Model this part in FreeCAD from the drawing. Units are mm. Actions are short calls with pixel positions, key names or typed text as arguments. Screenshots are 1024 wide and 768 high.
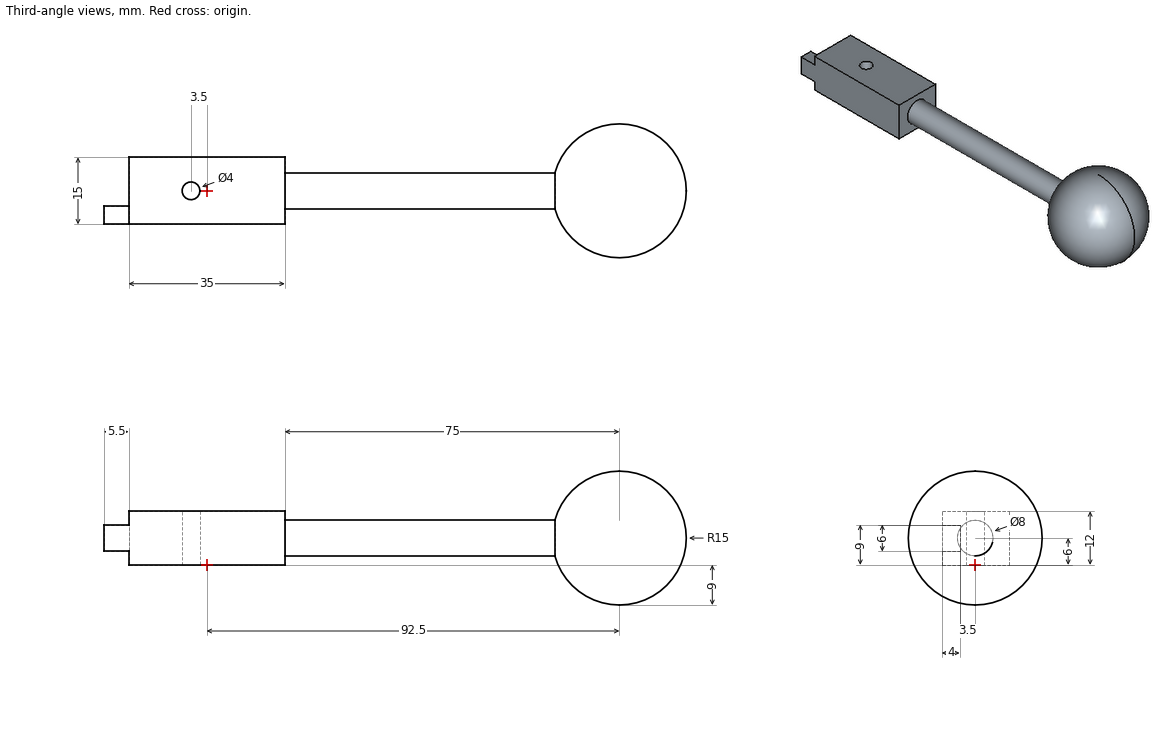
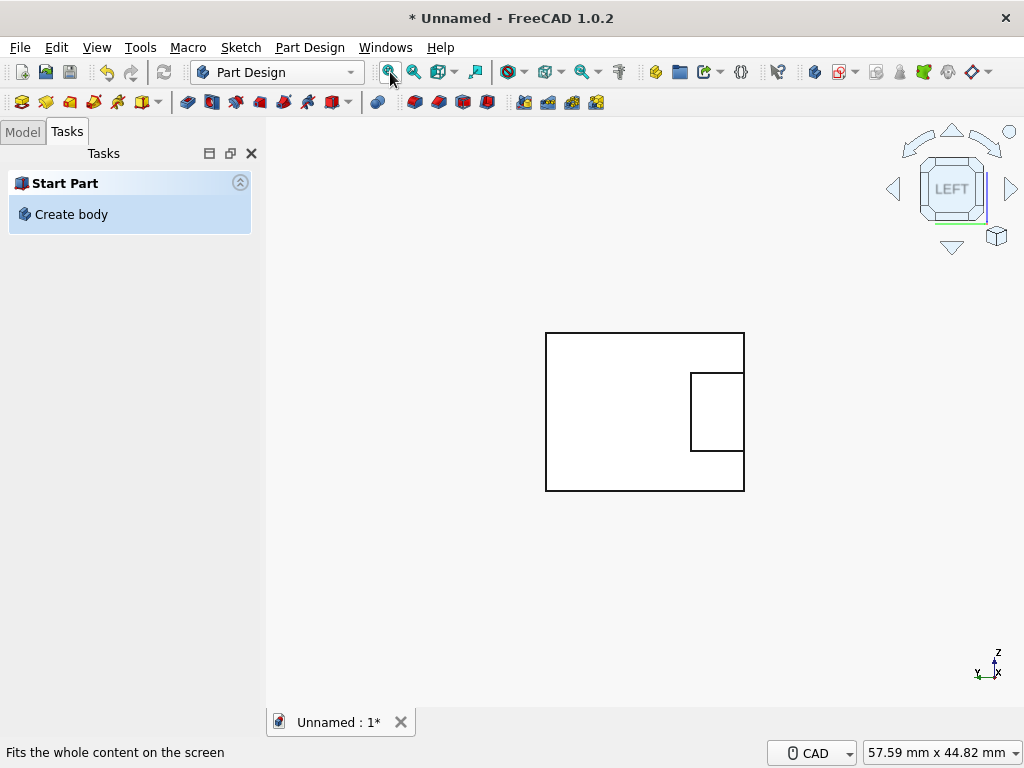
key(0)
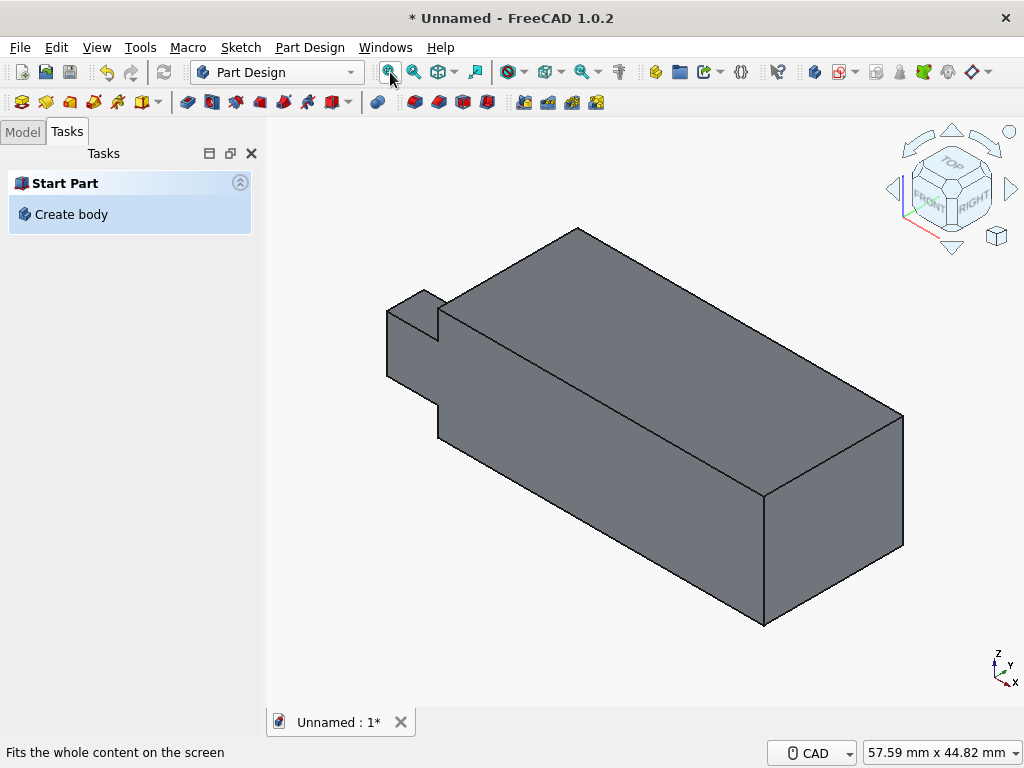
click(833, 520)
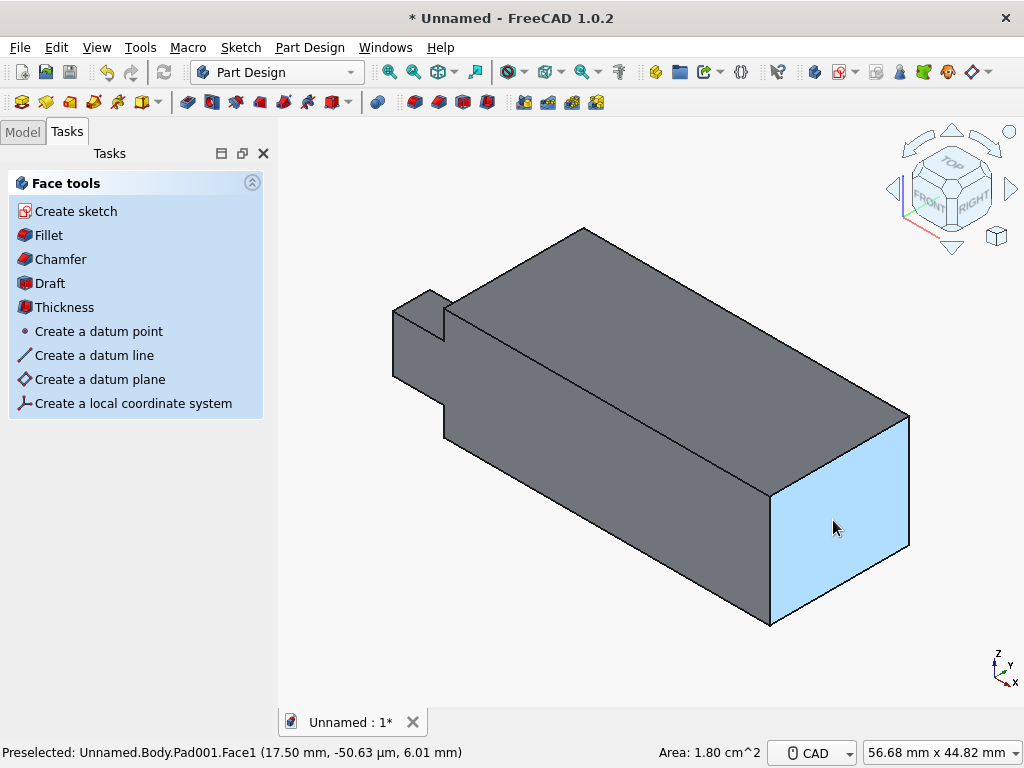
click(840, 72)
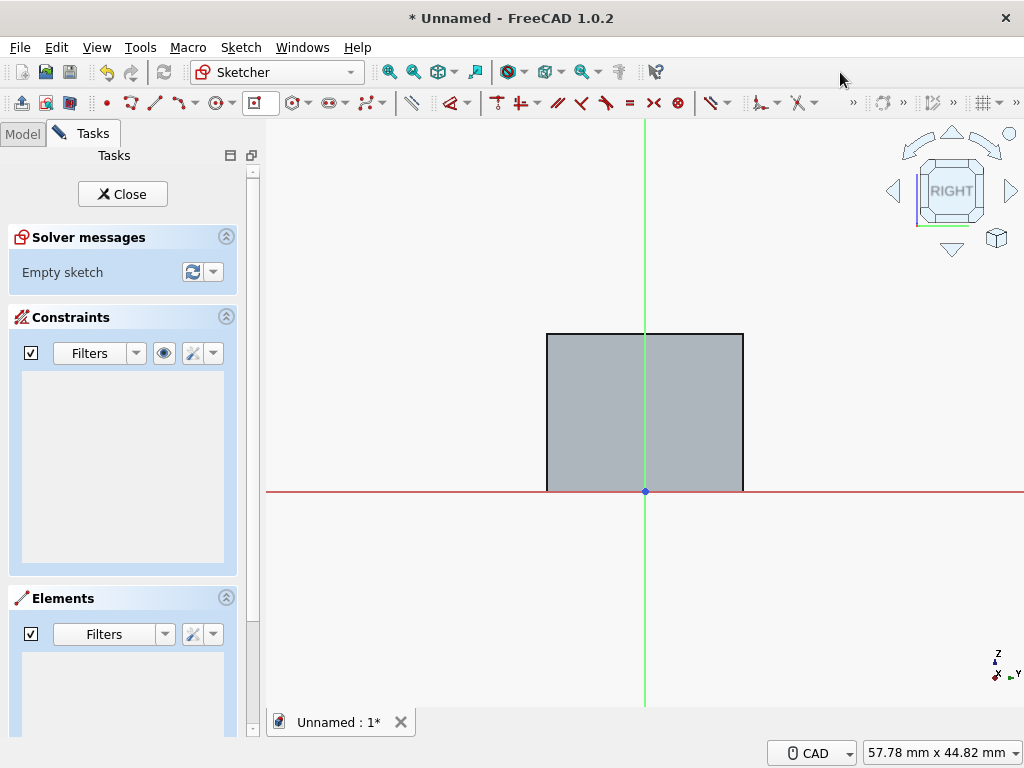
scroll(685, 434, up, 5)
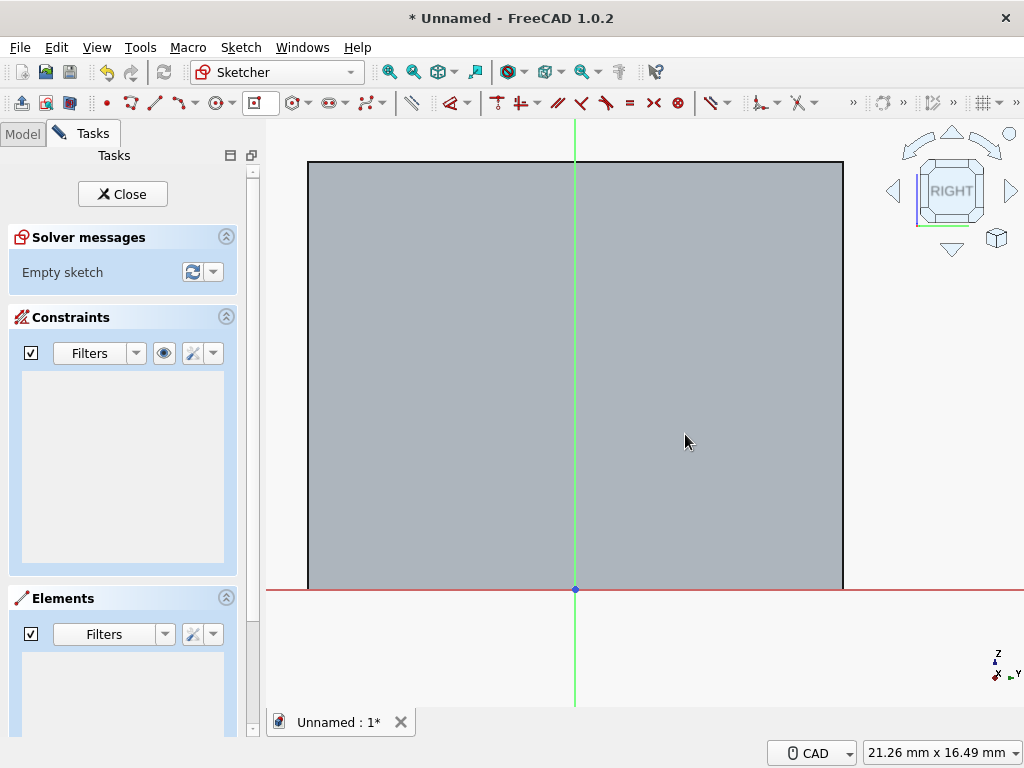
click(216, 104)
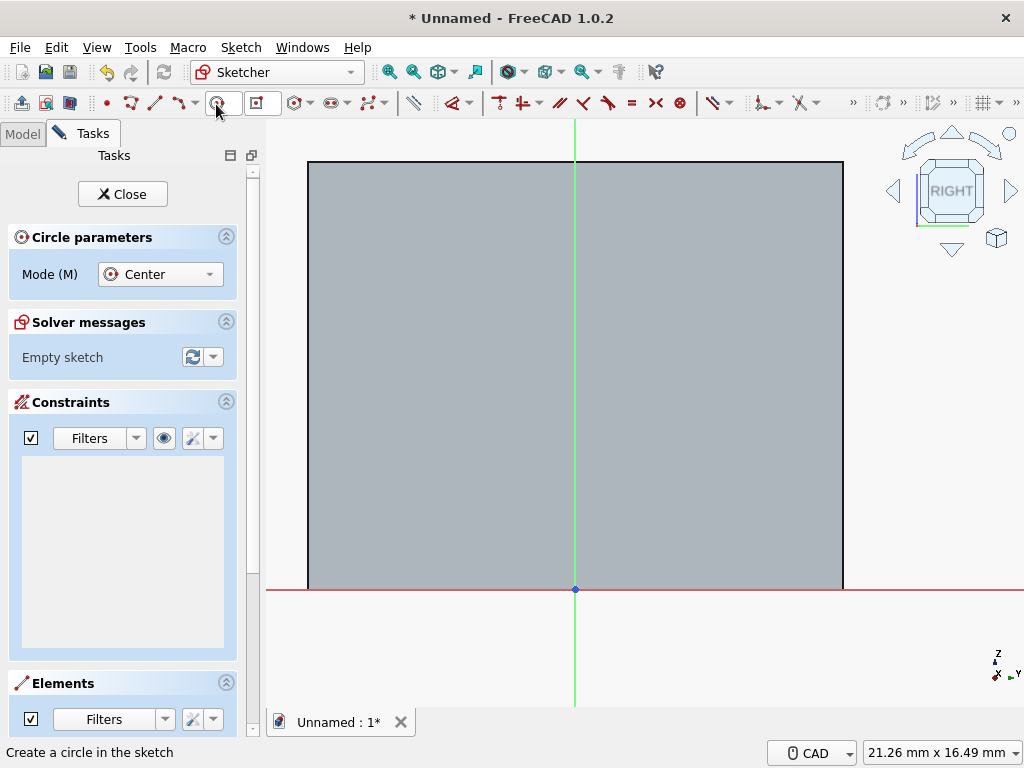
click(575, 376)
click(676, 275)
key(Escape)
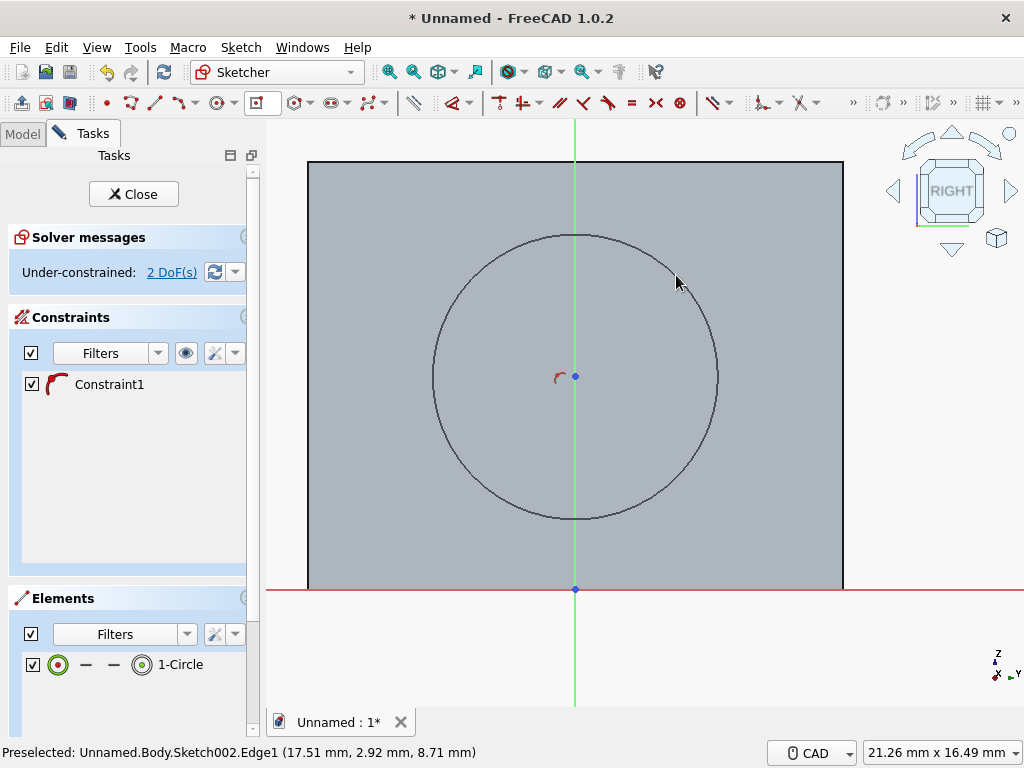
click(452, 104)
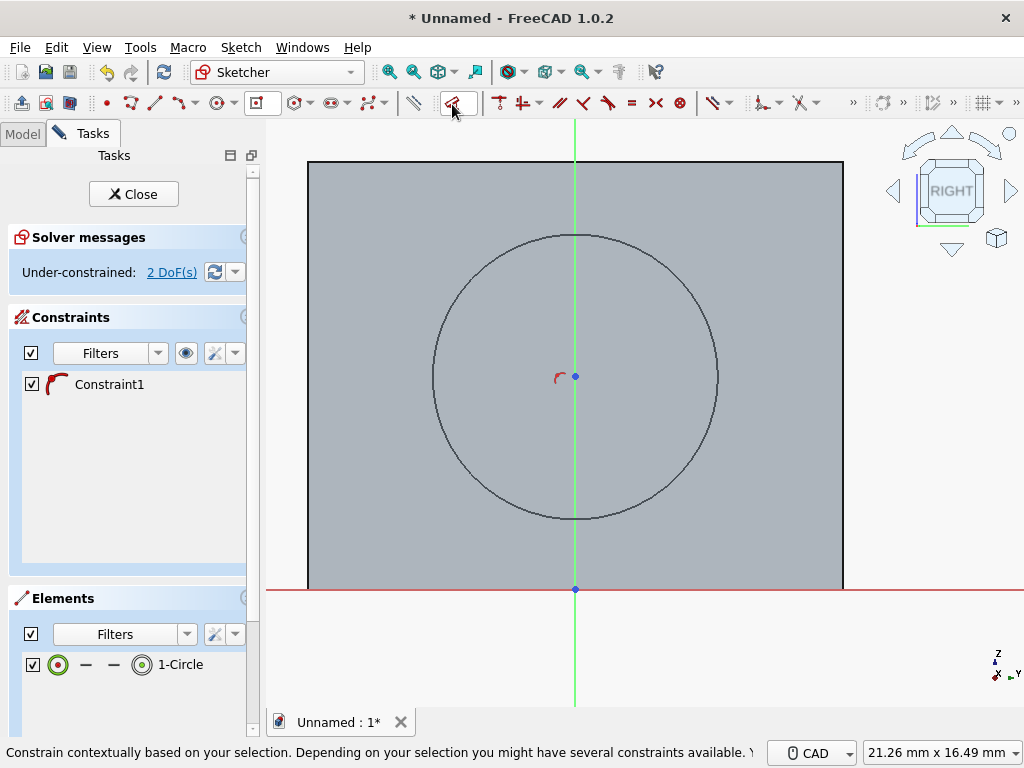
click(676, 276)
click(699, 253)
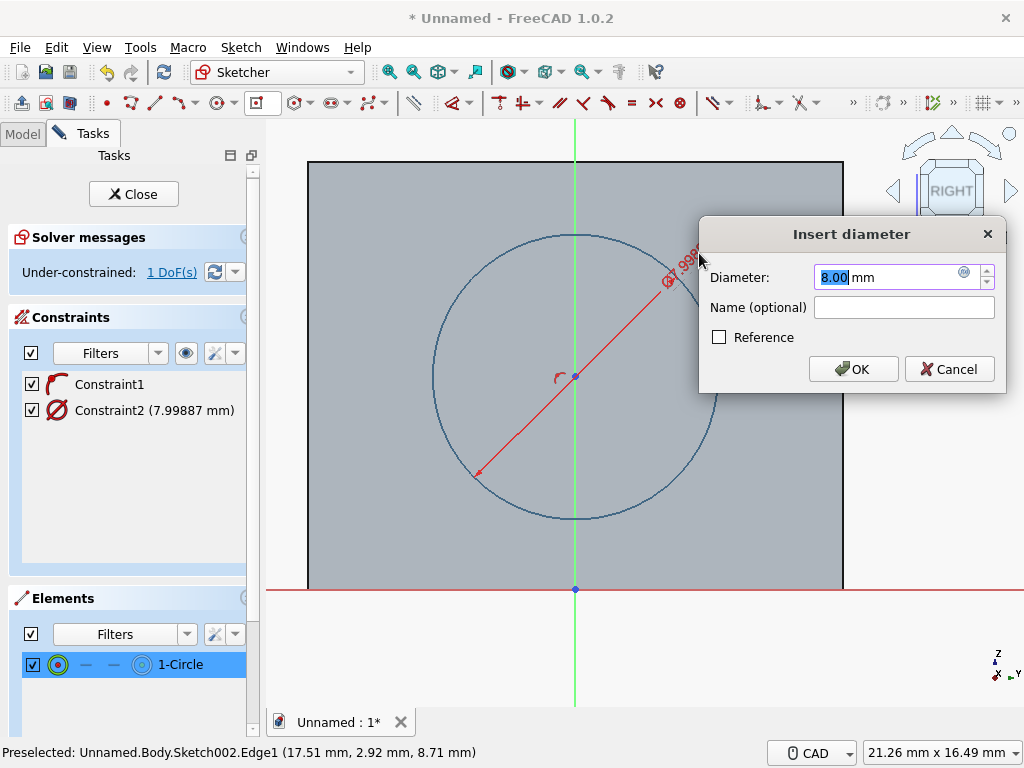
text(8)
key(Return)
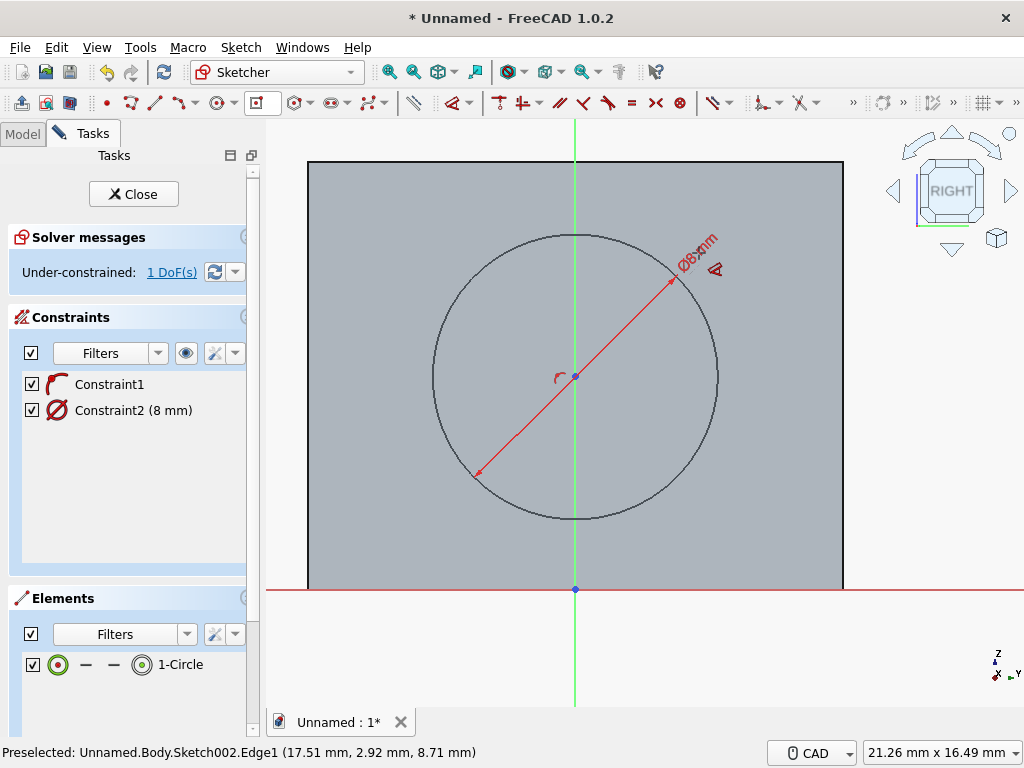
click(575, 377)
click(609, 483)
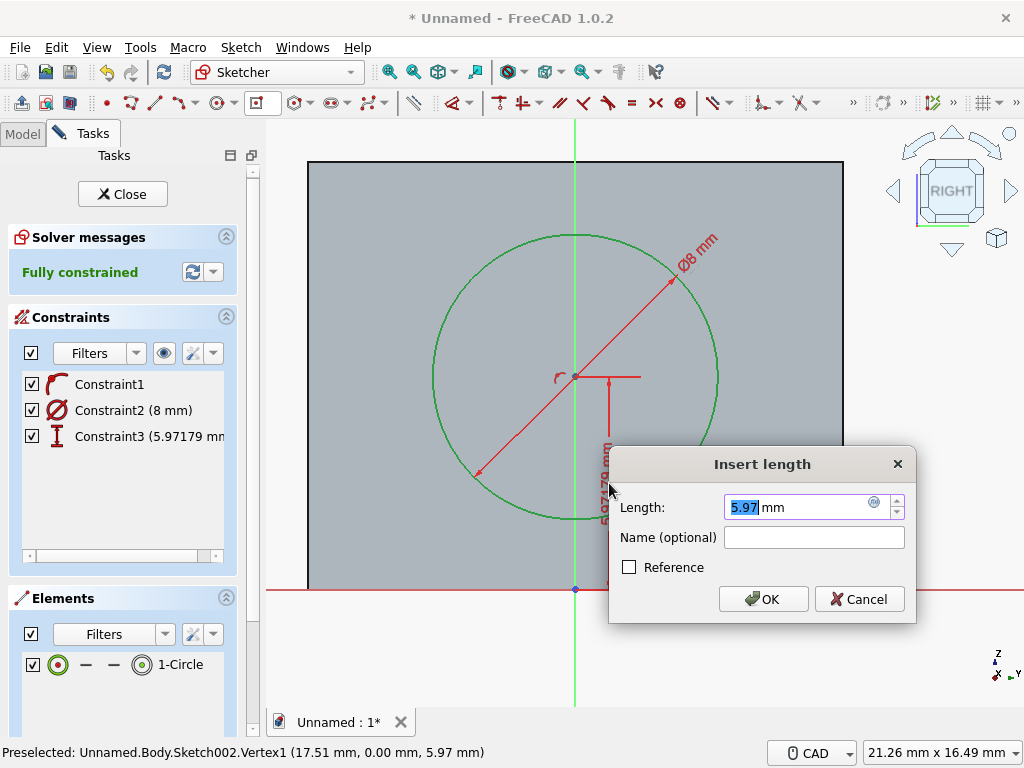
text(6)
key(Return)
key(Escape)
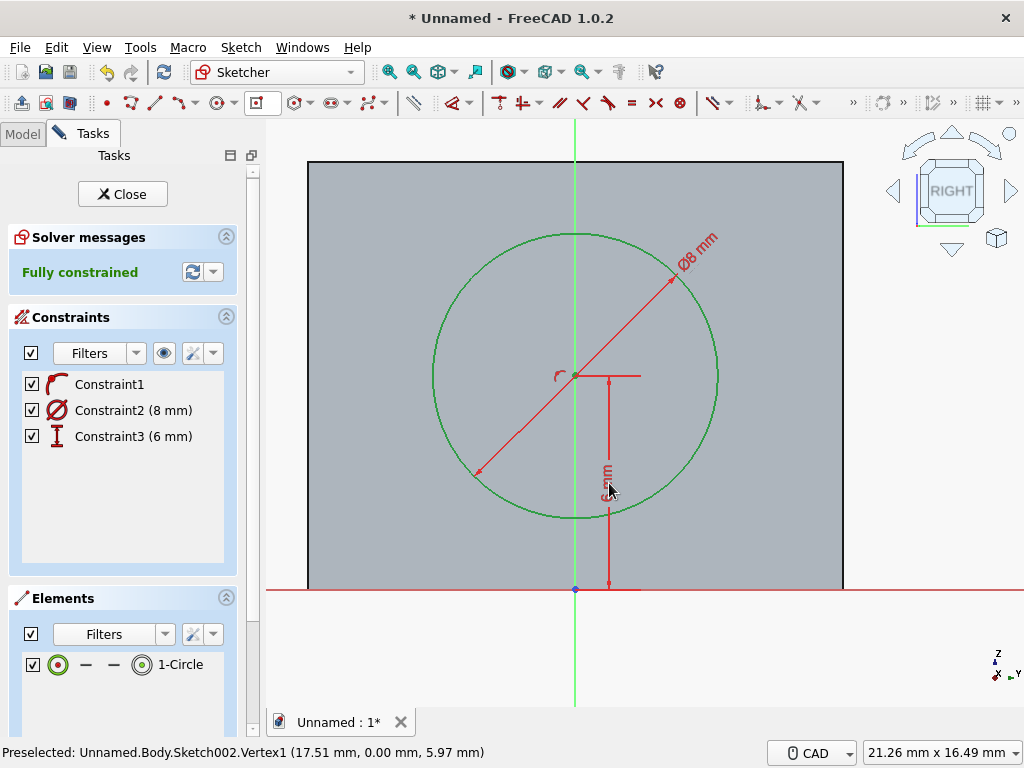
click(123, 194)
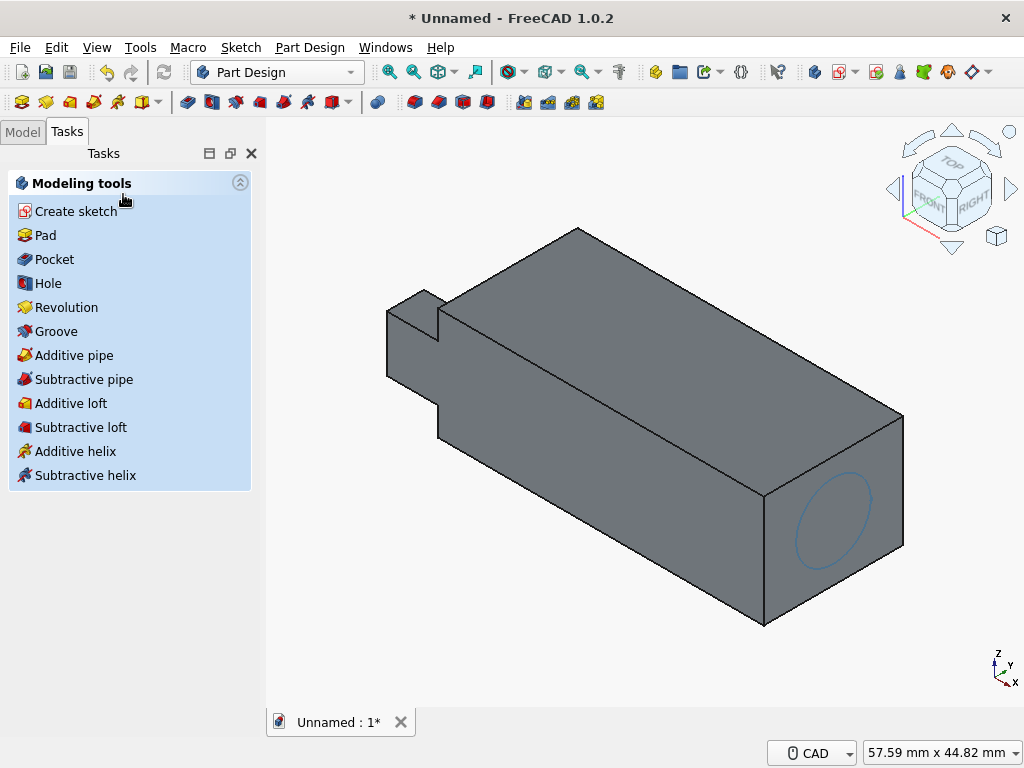
click(22, 102)